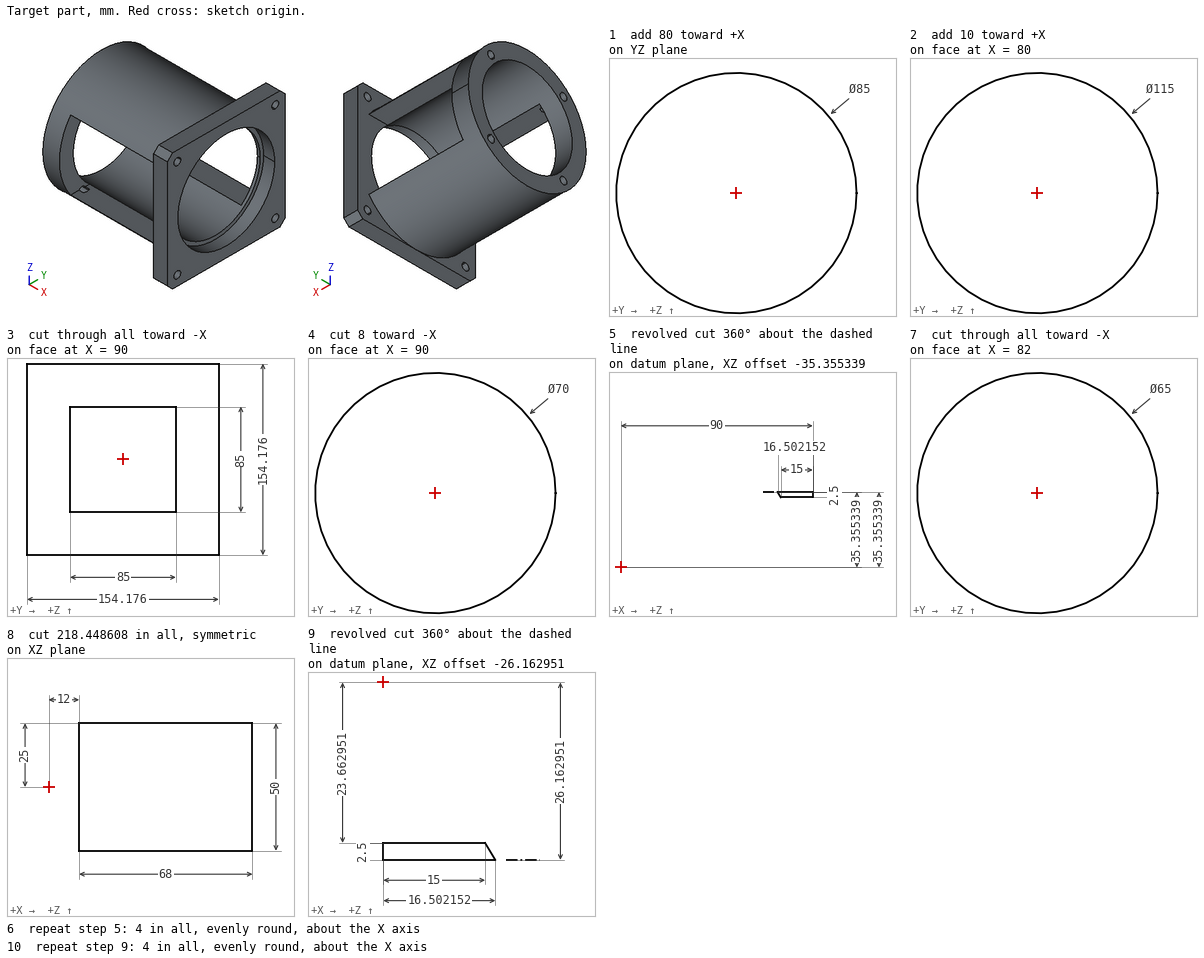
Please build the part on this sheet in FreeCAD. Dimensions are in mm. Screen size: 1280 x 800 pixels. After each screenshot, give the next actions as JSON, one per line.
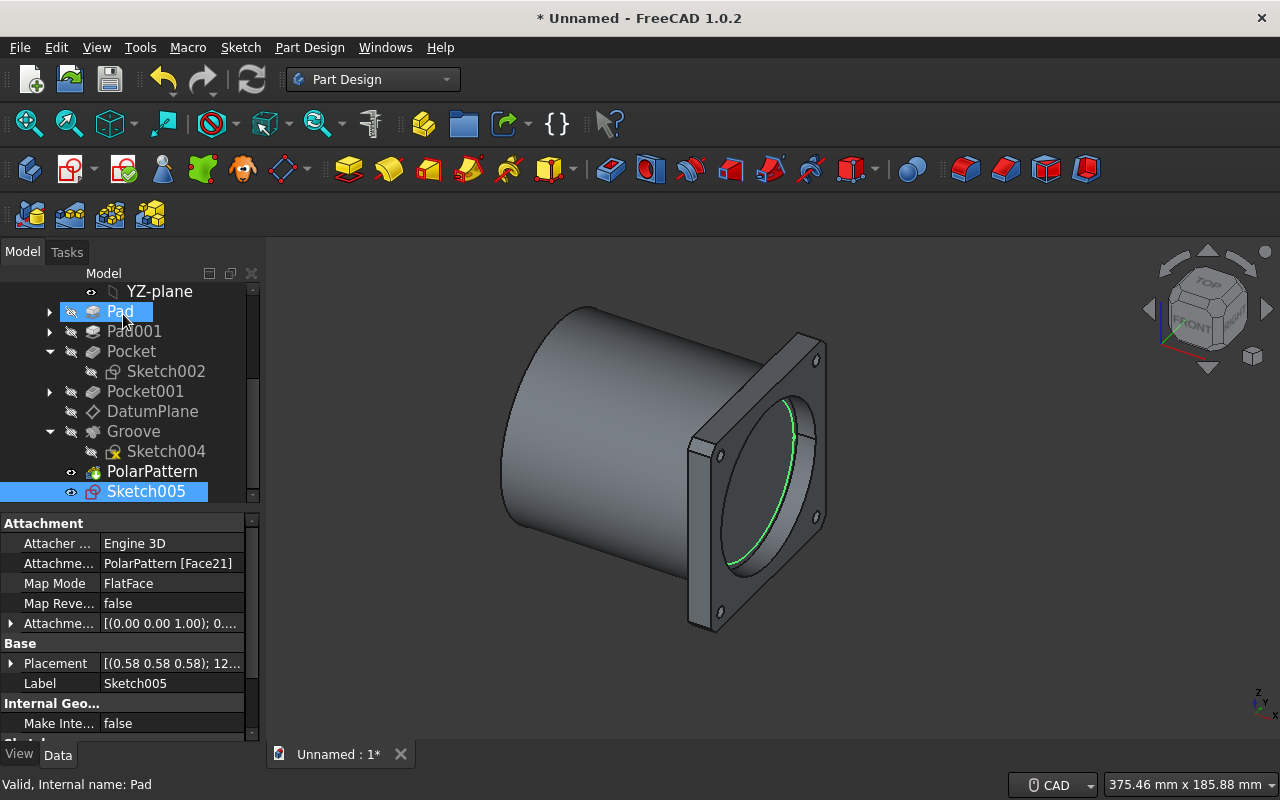
{"action": "left_click", "coordinate": [612, 170]}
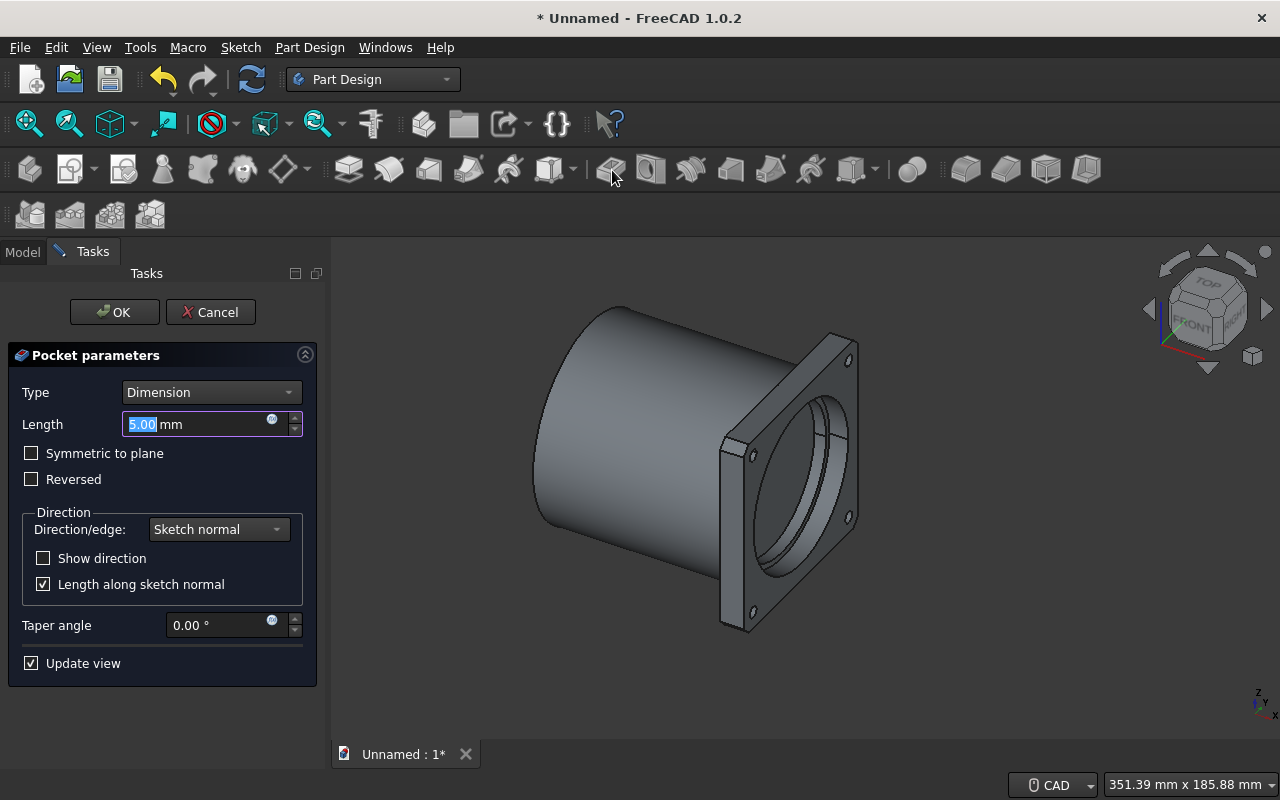
{"action": "left_click", "coordinate": [212, 392]}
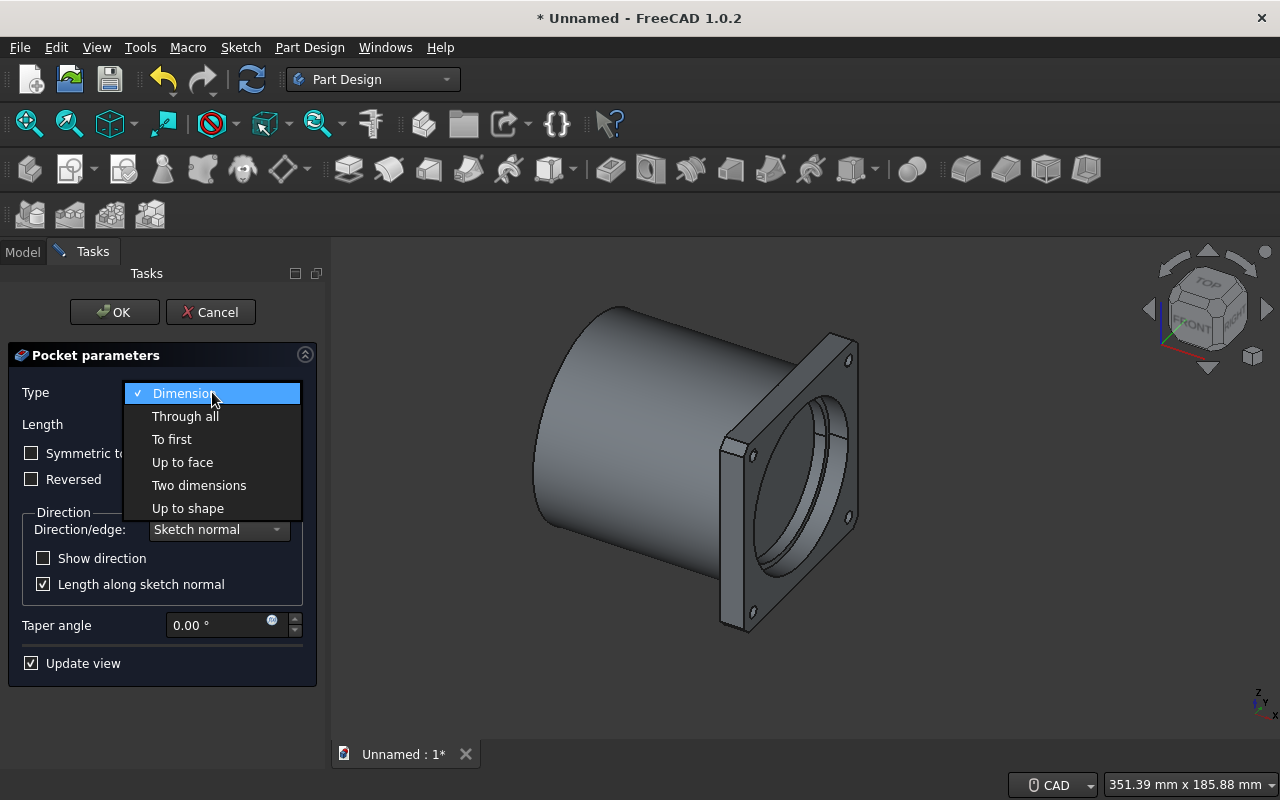
{"action": "left_click", "coordinate": [212, 416]}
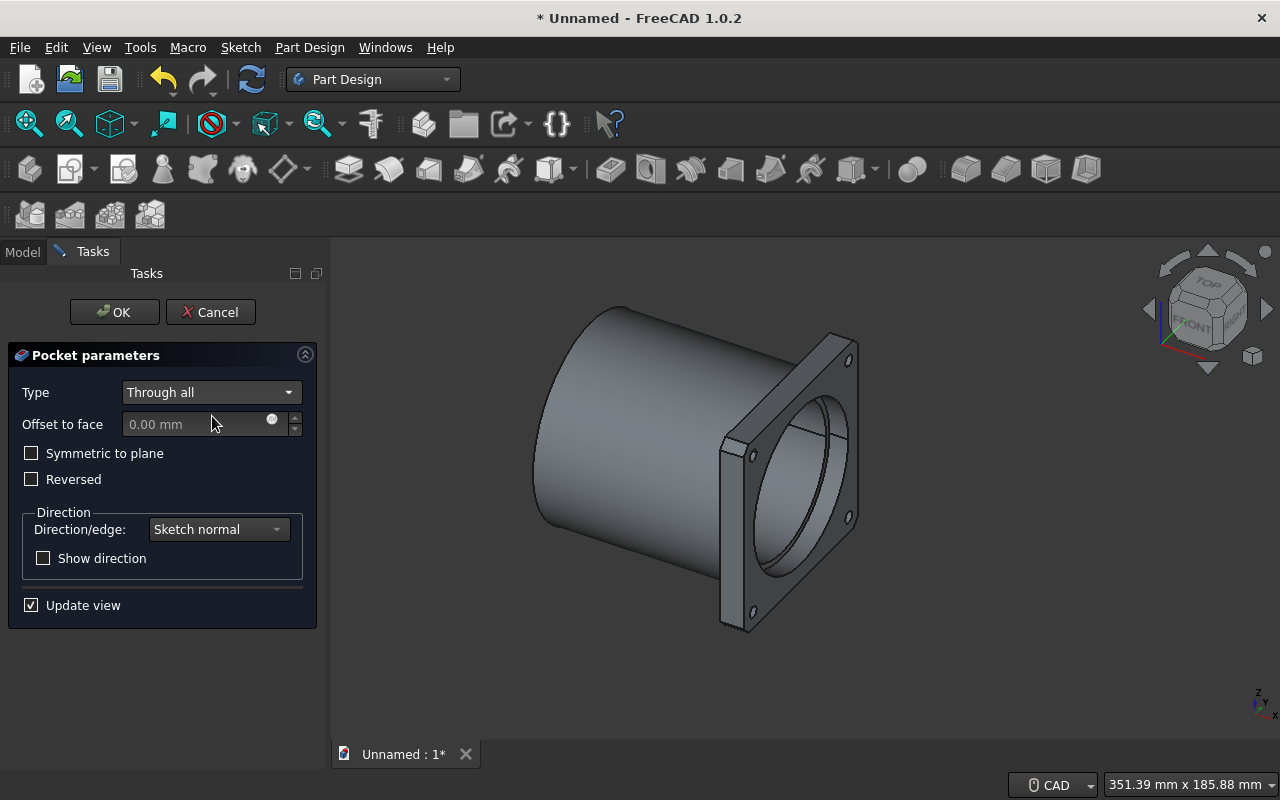
{"action": "left_click", "coordinate": [115, 312]}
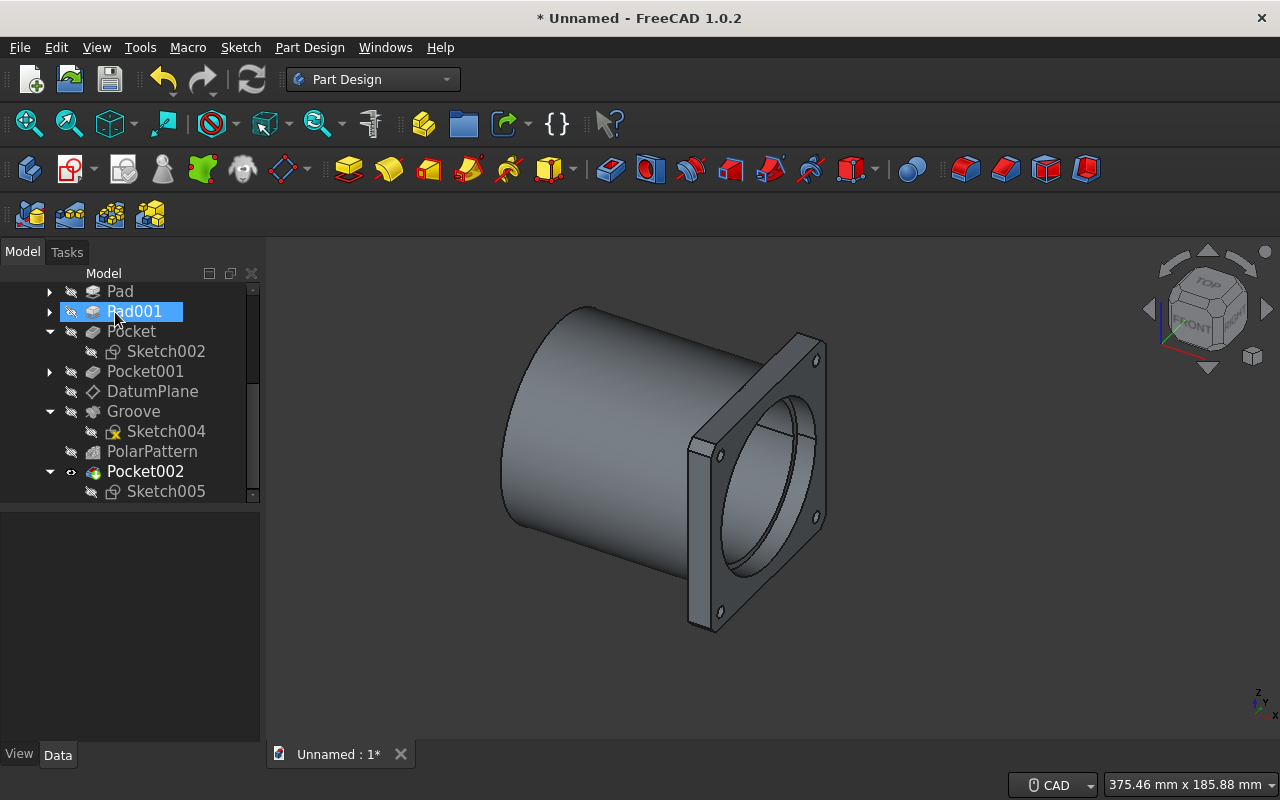
{"action": "left_click", "coordinate": [70, 170]}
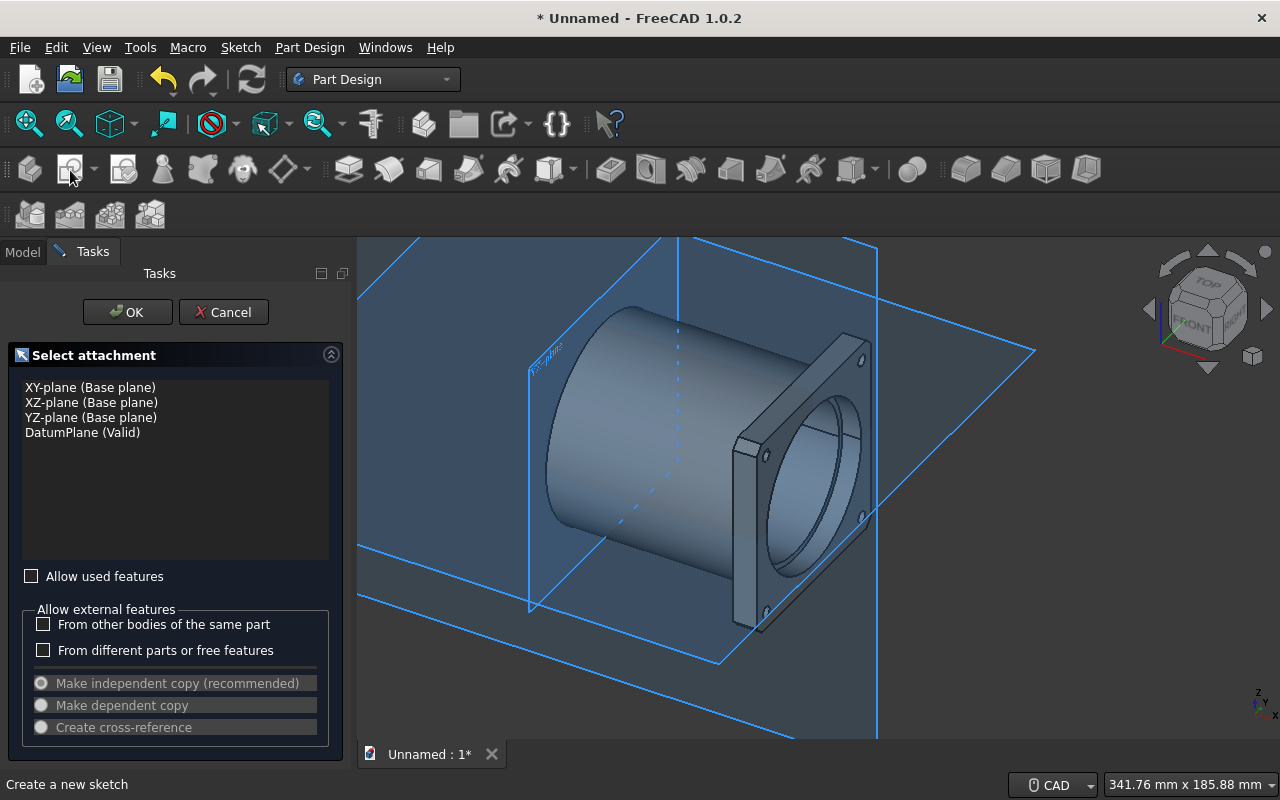
{"action": "left_click", "coordinate": [82, 402]}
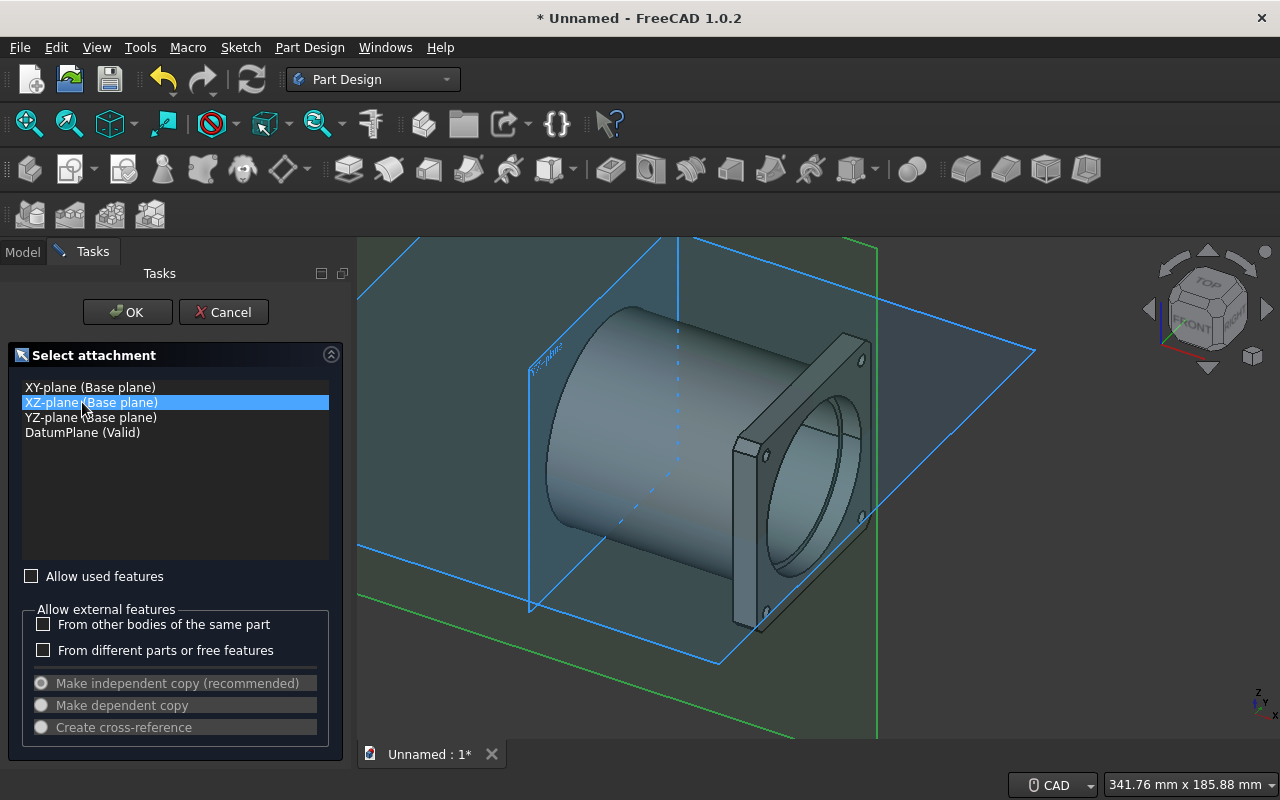
{"action": "left_click", "coordinate": [128, 312]}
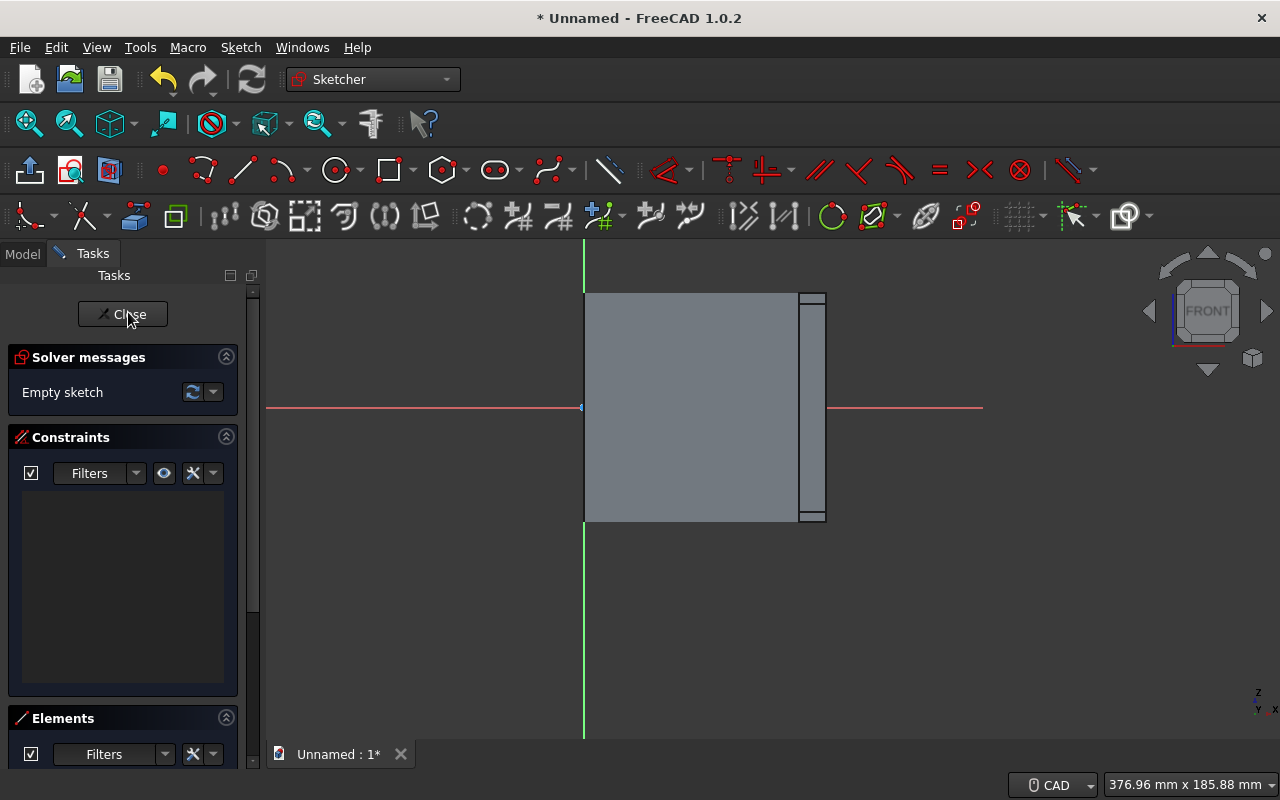
{"action": "left_click", "coordinate": [110, 170]}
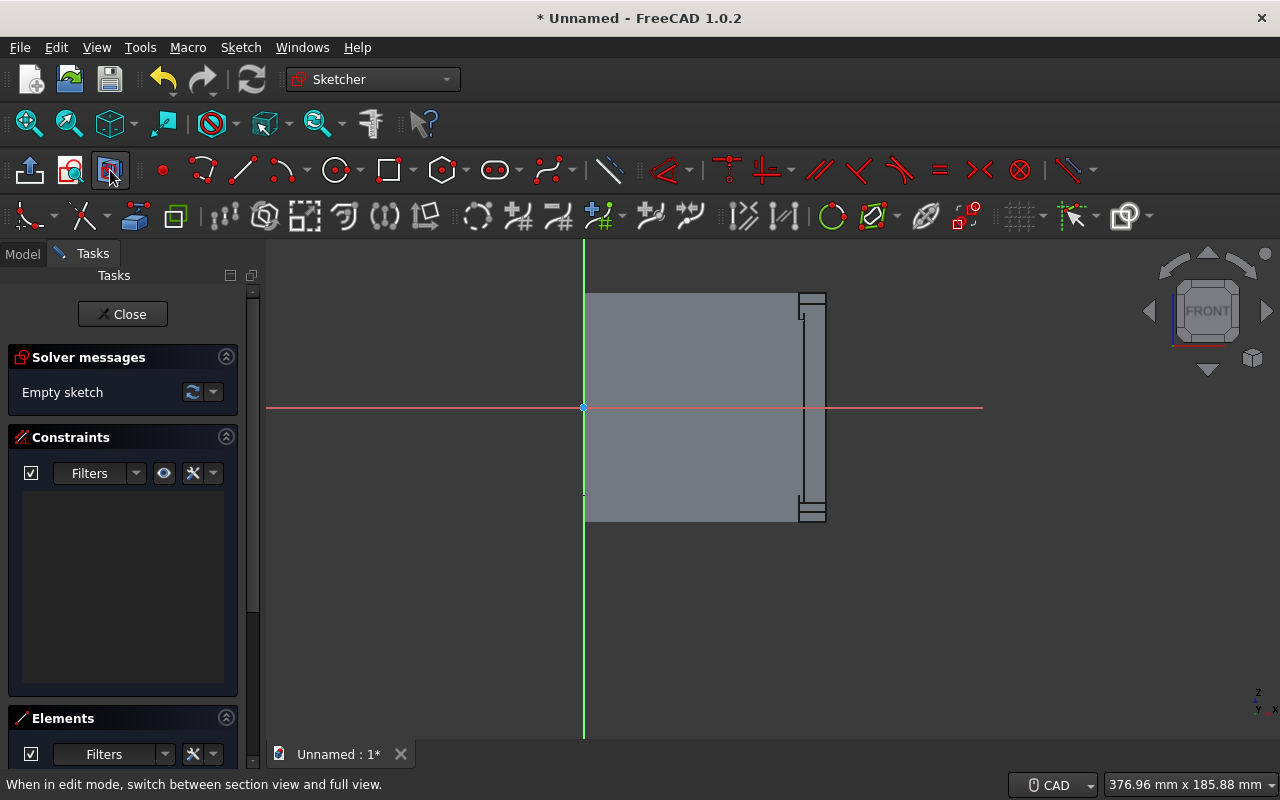
{"action": "scroll", "coordinate": [680, 342], "scroll_direction": "up", "scroll_amount": 4}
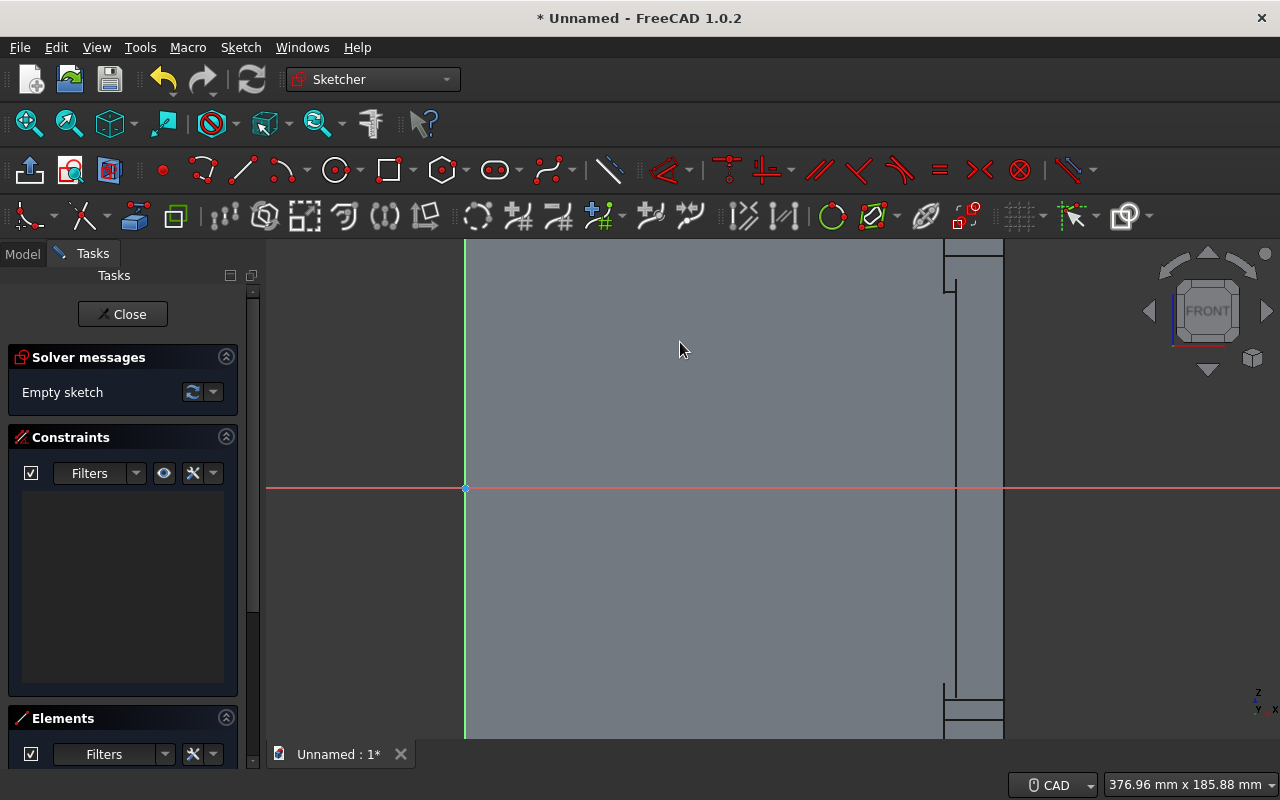
{"action": "left_click", "coordinate": [390, 170]}